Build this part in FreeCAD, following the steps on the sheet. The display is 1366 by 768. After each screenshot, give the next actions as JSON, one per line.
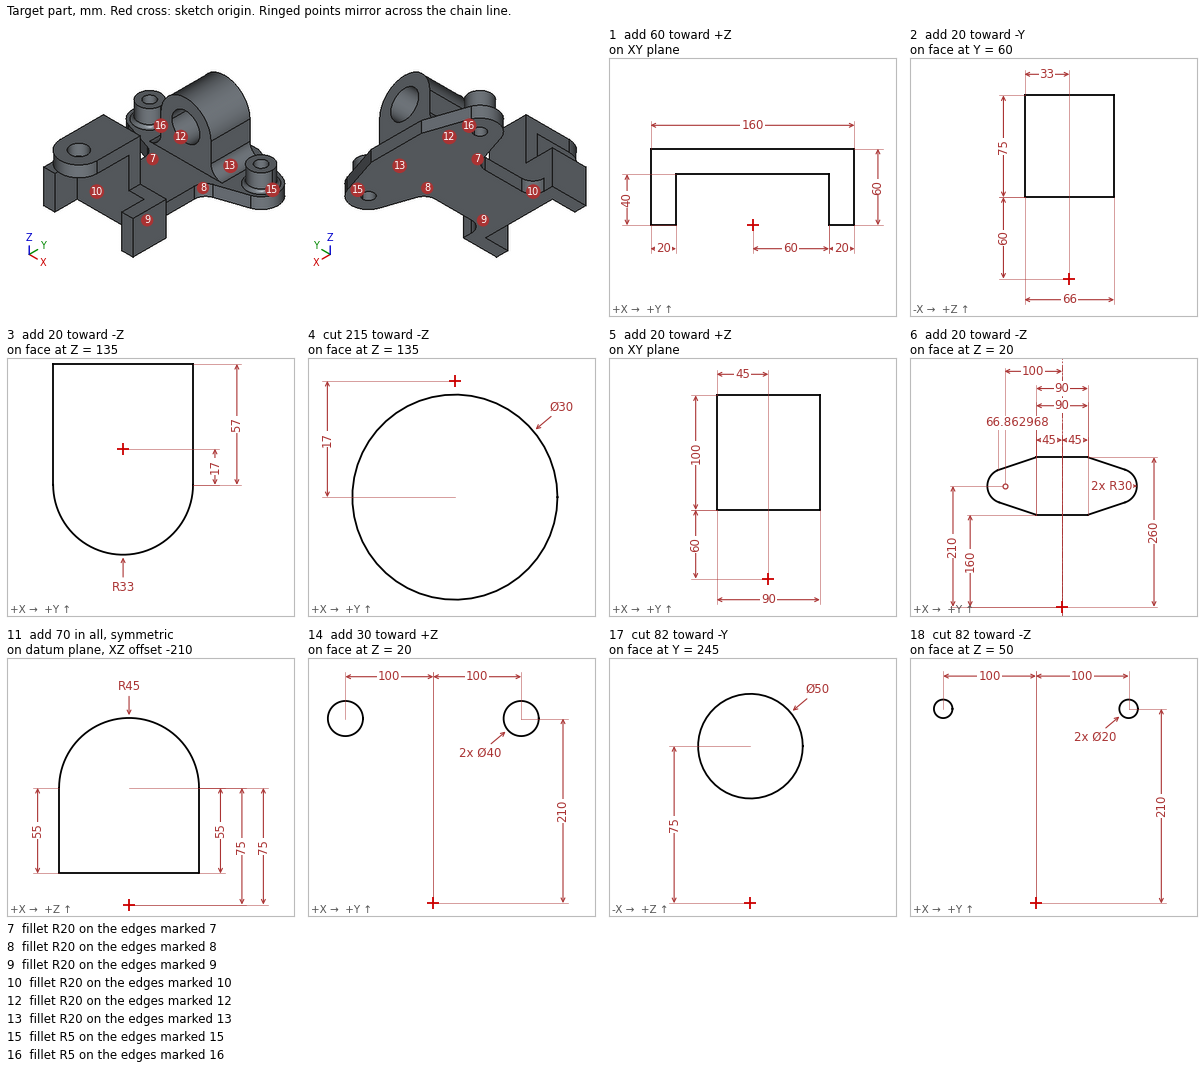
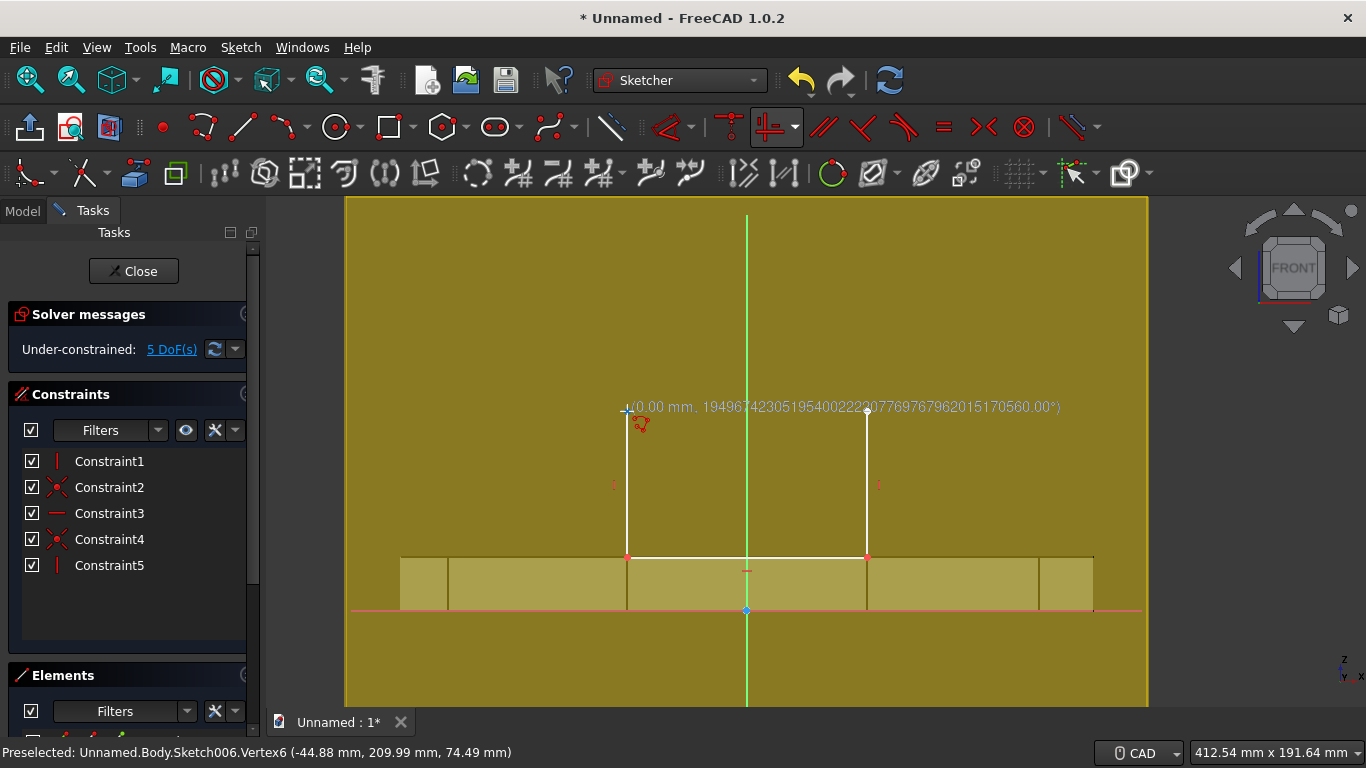
{"action": "key", "text": "g 3 a"}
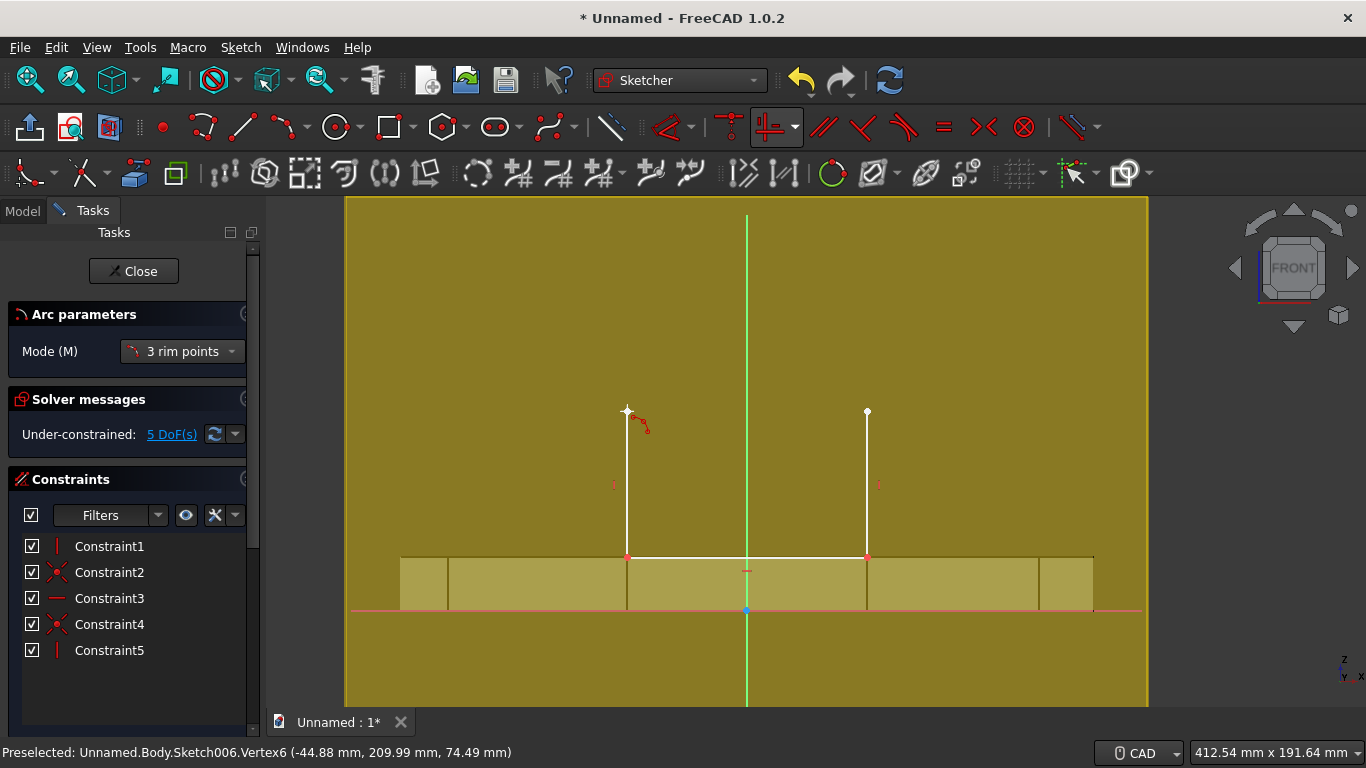
{"action": "left_click", "coordinate": [627, 412]}
{"action": "left_click", "coordinate": [867, 412]}
{"action": "left_click", "coordinate": [784, 297]}
{"action": "key", "text": "Escape"}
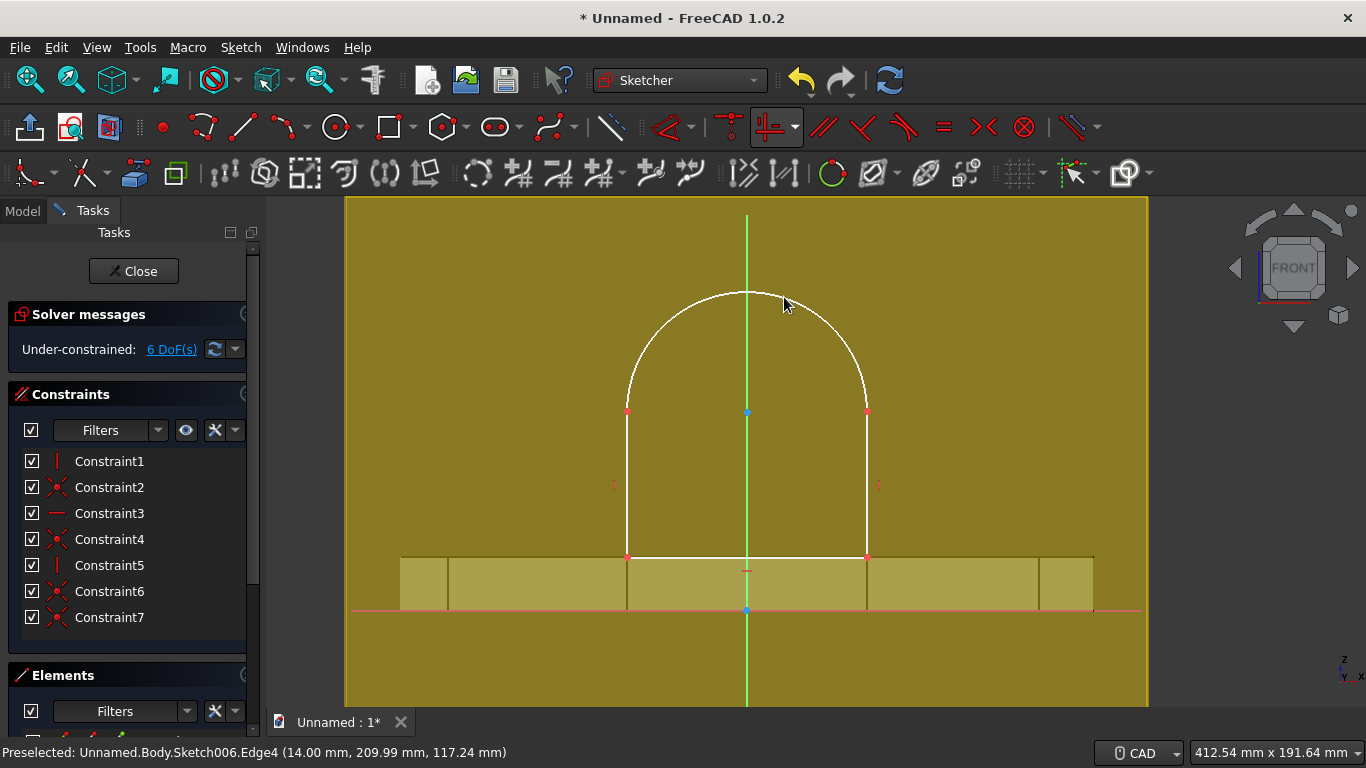
{"action": "left_click", "coordinate": [747, 412]}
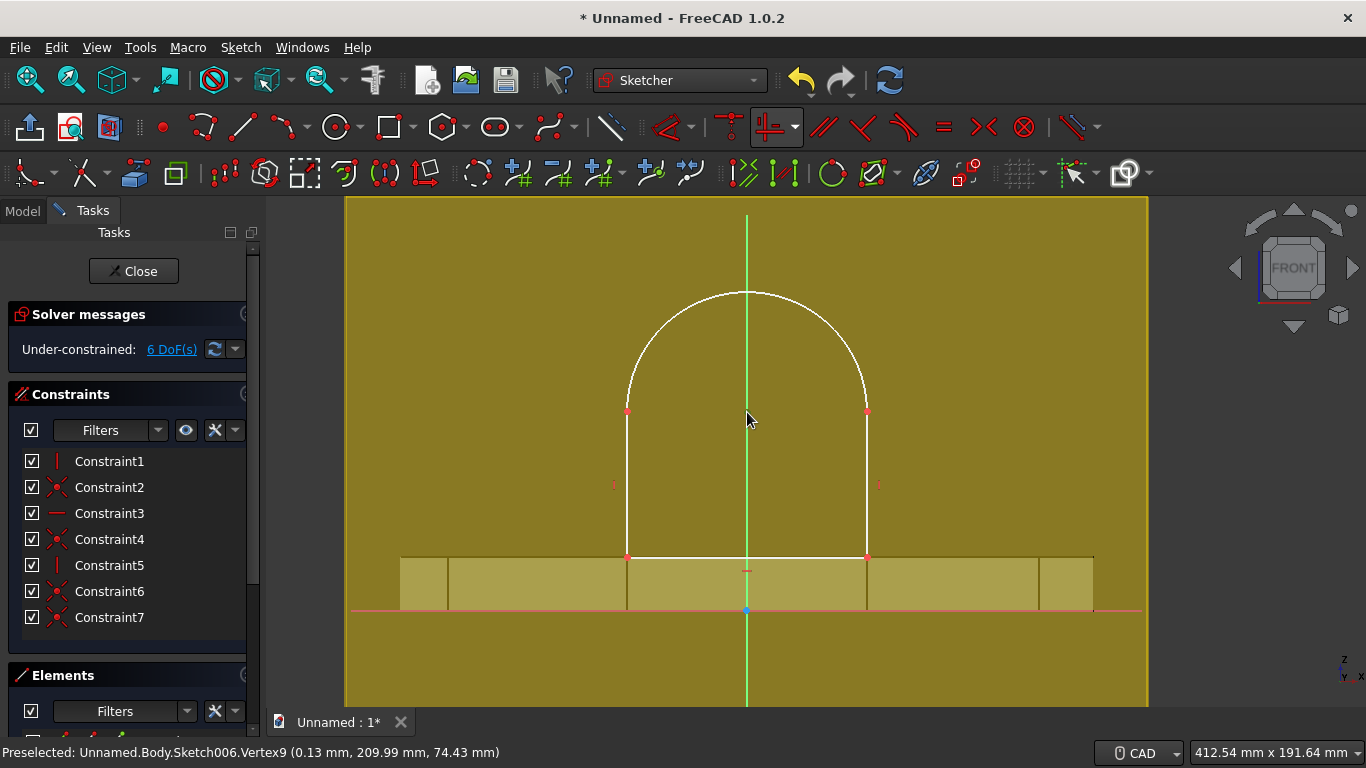
{"action": "left_click", "coordinate": [747, 646]}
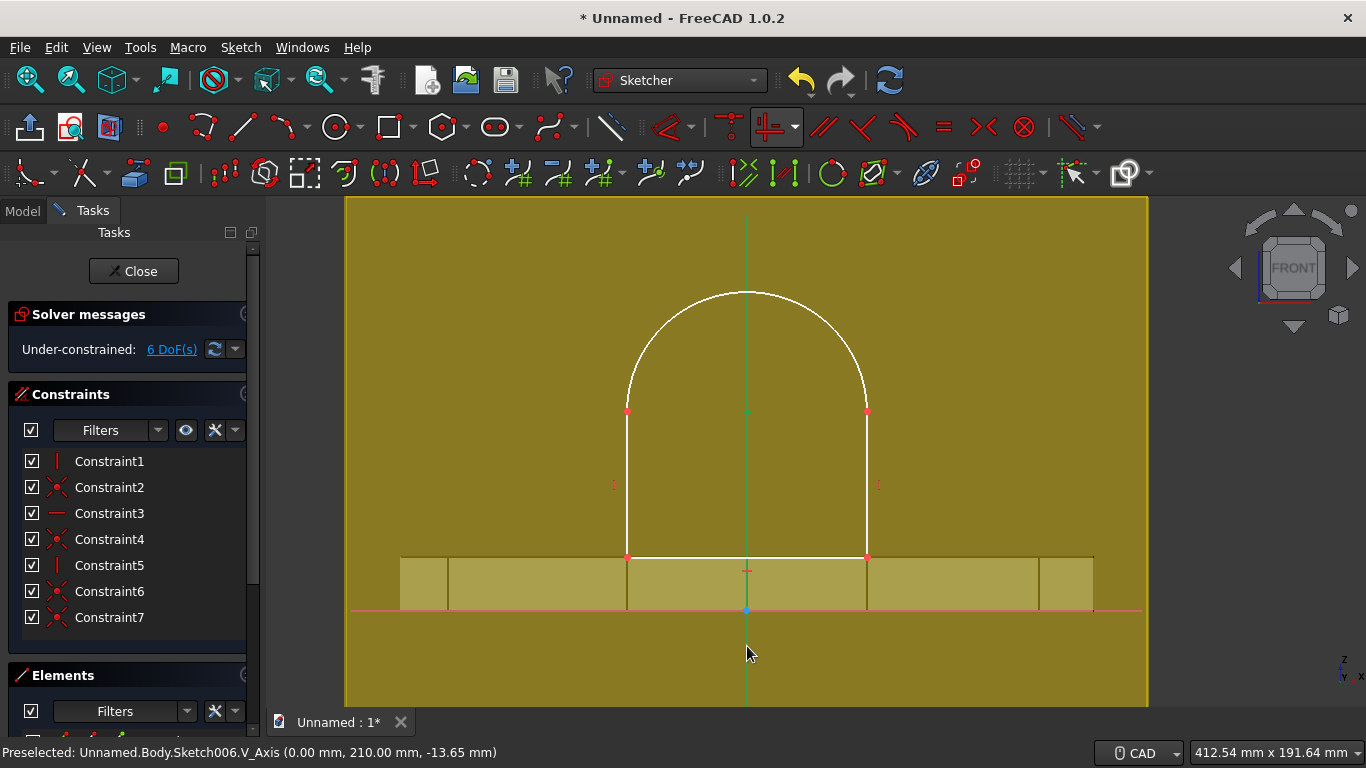
{"action": "key", "text": "c"}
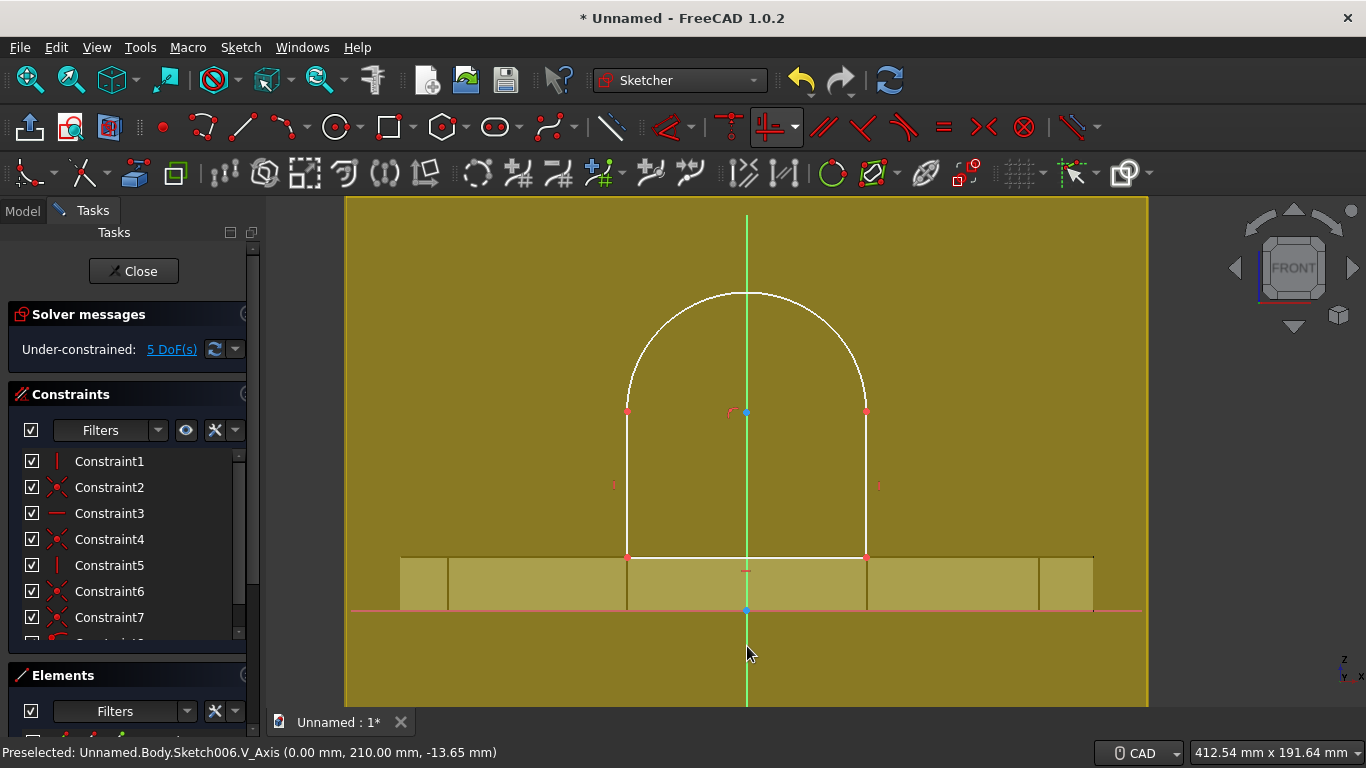
{"action": "key", "text": "d"}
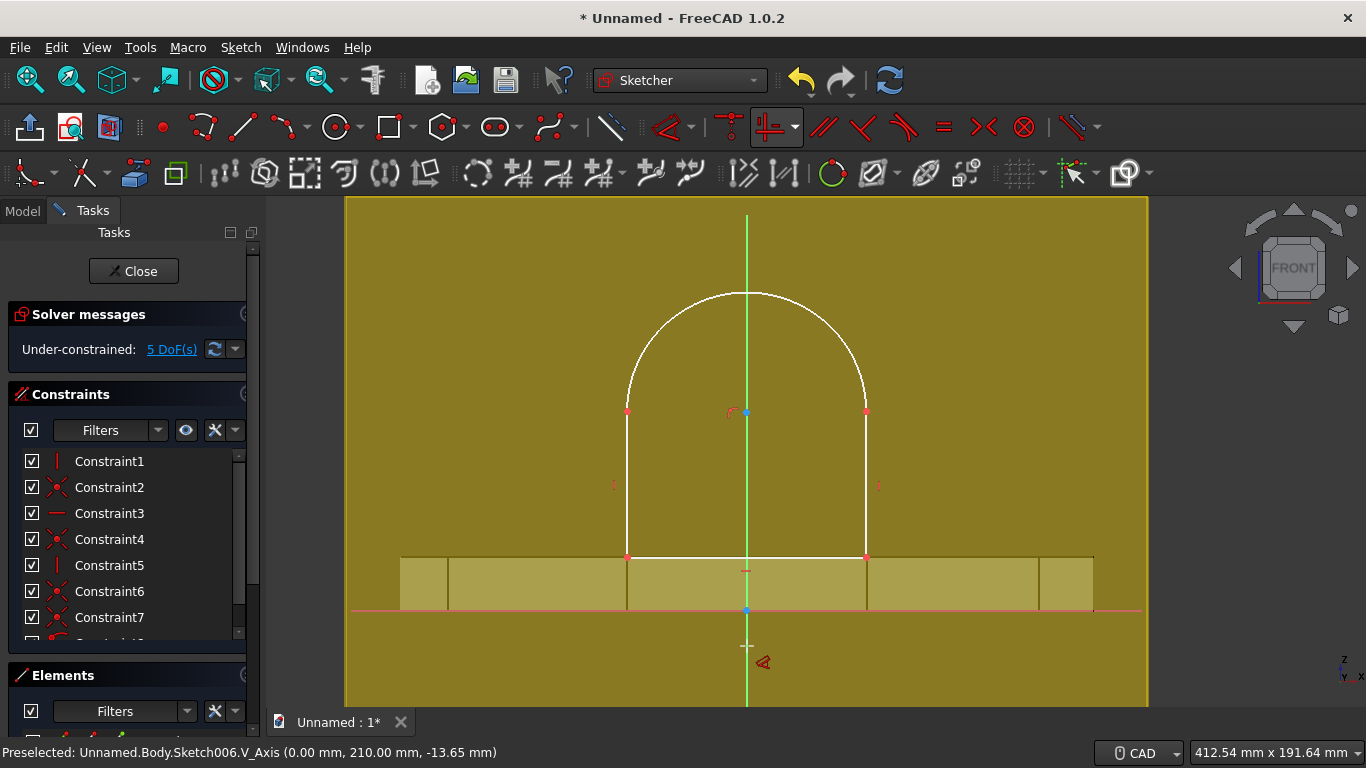
{"action": "left_click", "coordinate": [817, 315]}
{"action": "left_click", "coordinate": [836, 289]}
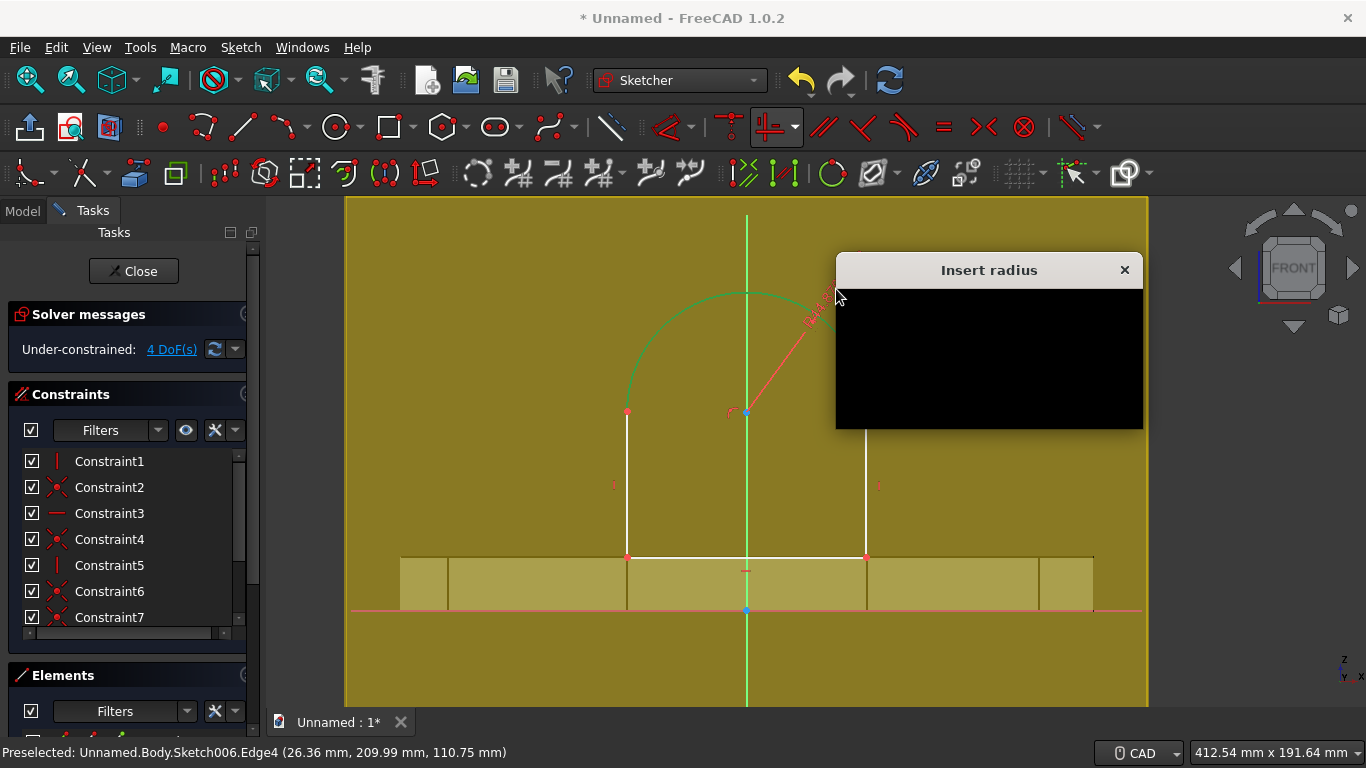
{"action": "type", "text": "45"}
{"action": "key", "text": "Return"}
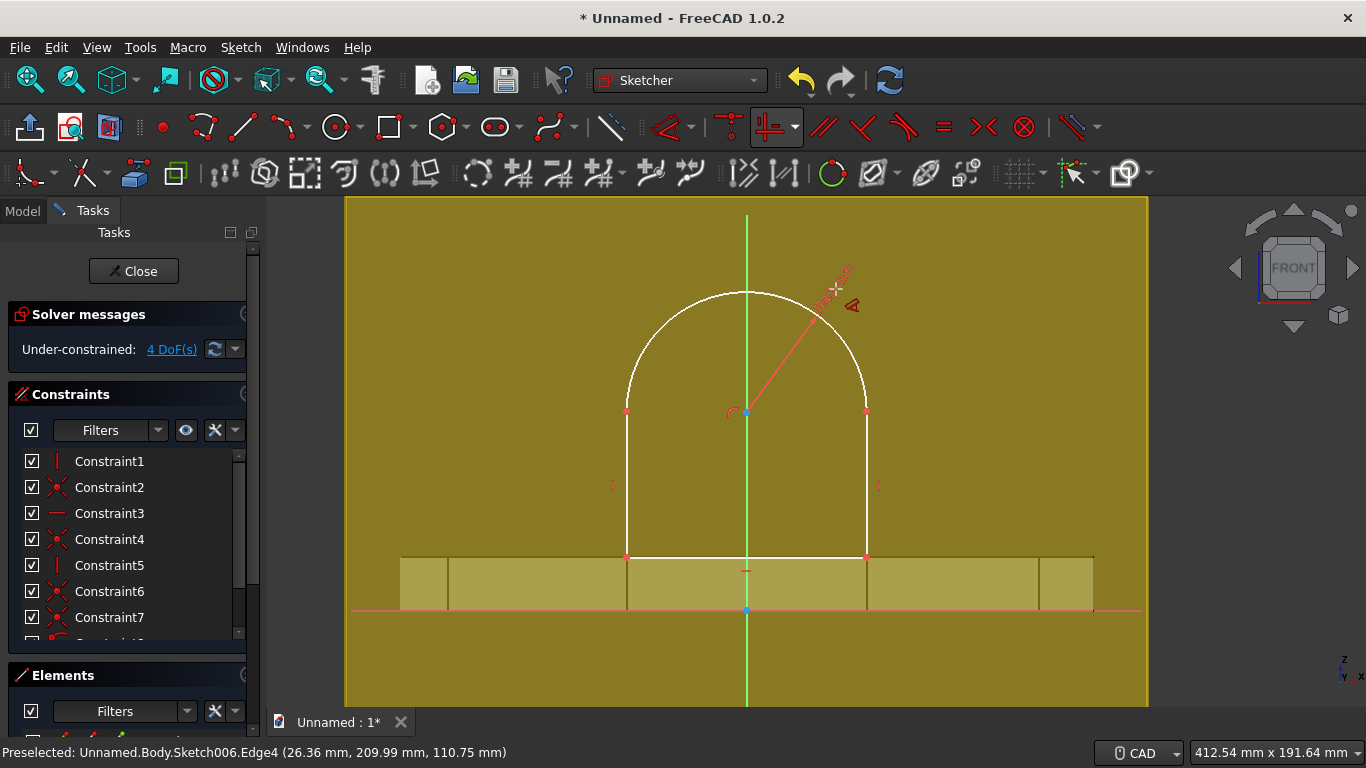
{"action": "left_click", "coordinate": [867, 456]}
{"action": "left_click", "coordinate": [901, 485]}